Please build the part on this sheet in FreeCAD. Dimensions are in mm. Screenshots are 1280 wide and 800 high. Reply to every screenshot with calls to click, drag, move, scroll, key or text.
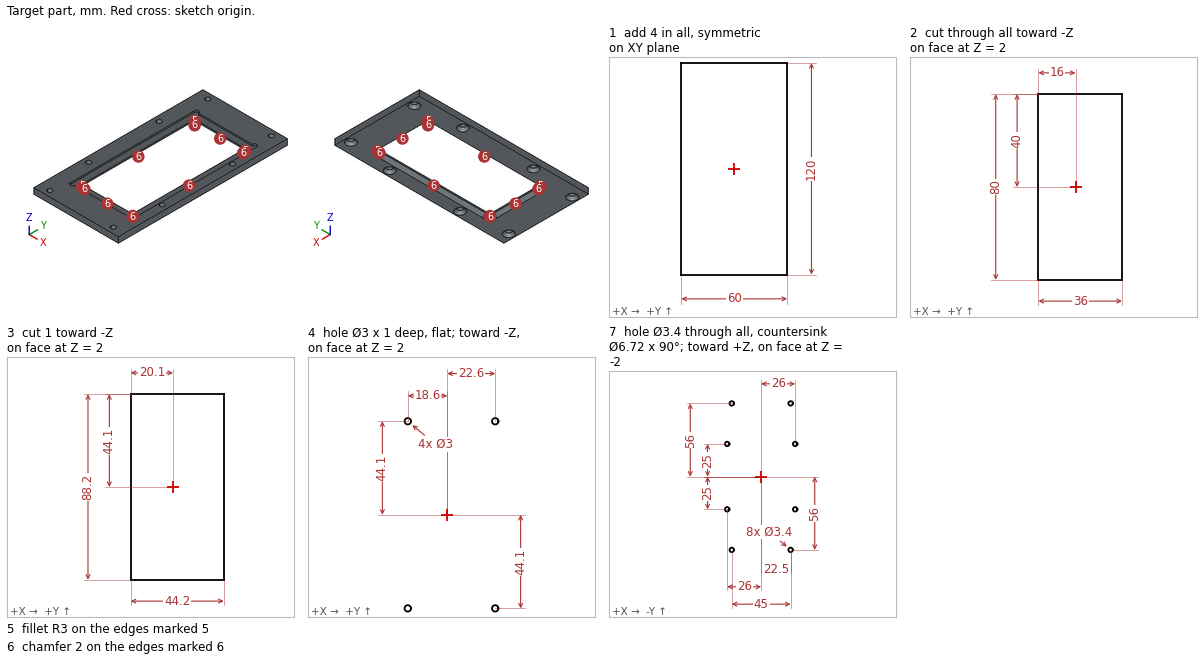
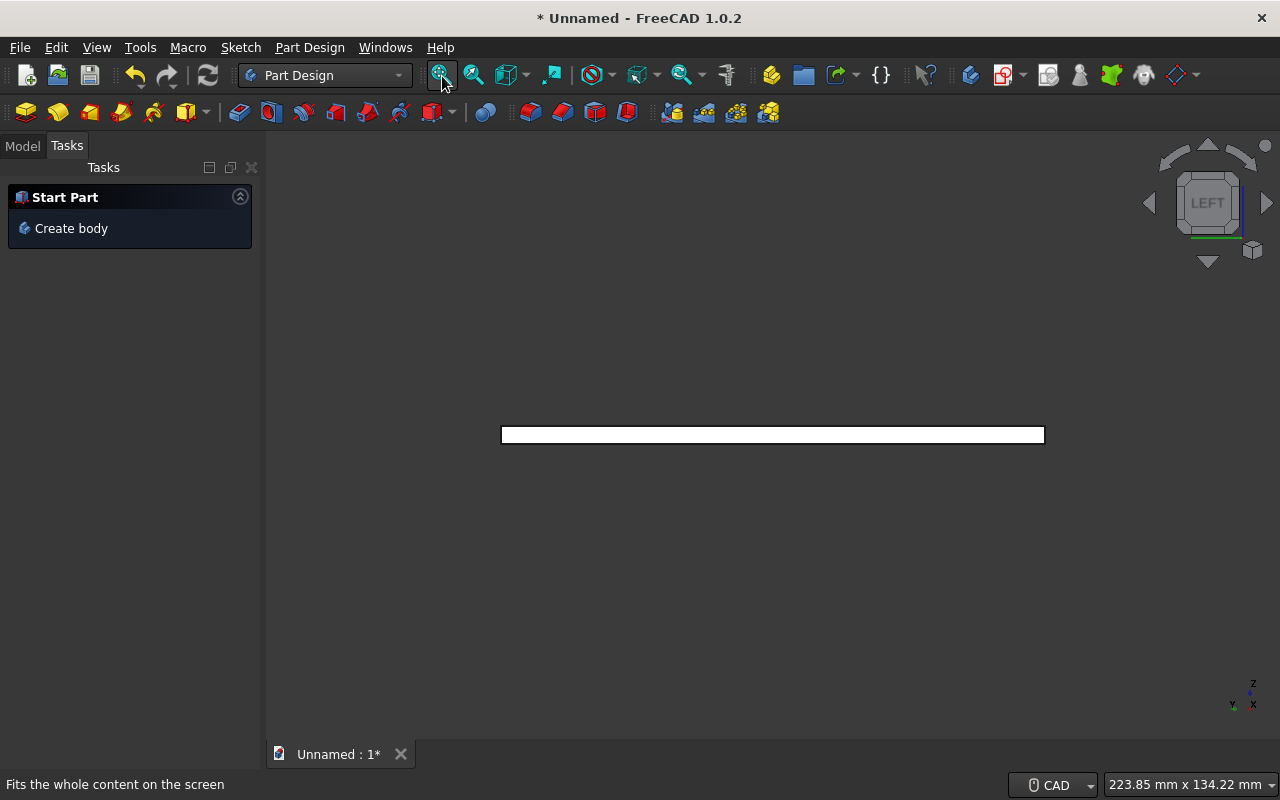
scroll(954, 436, up, 6)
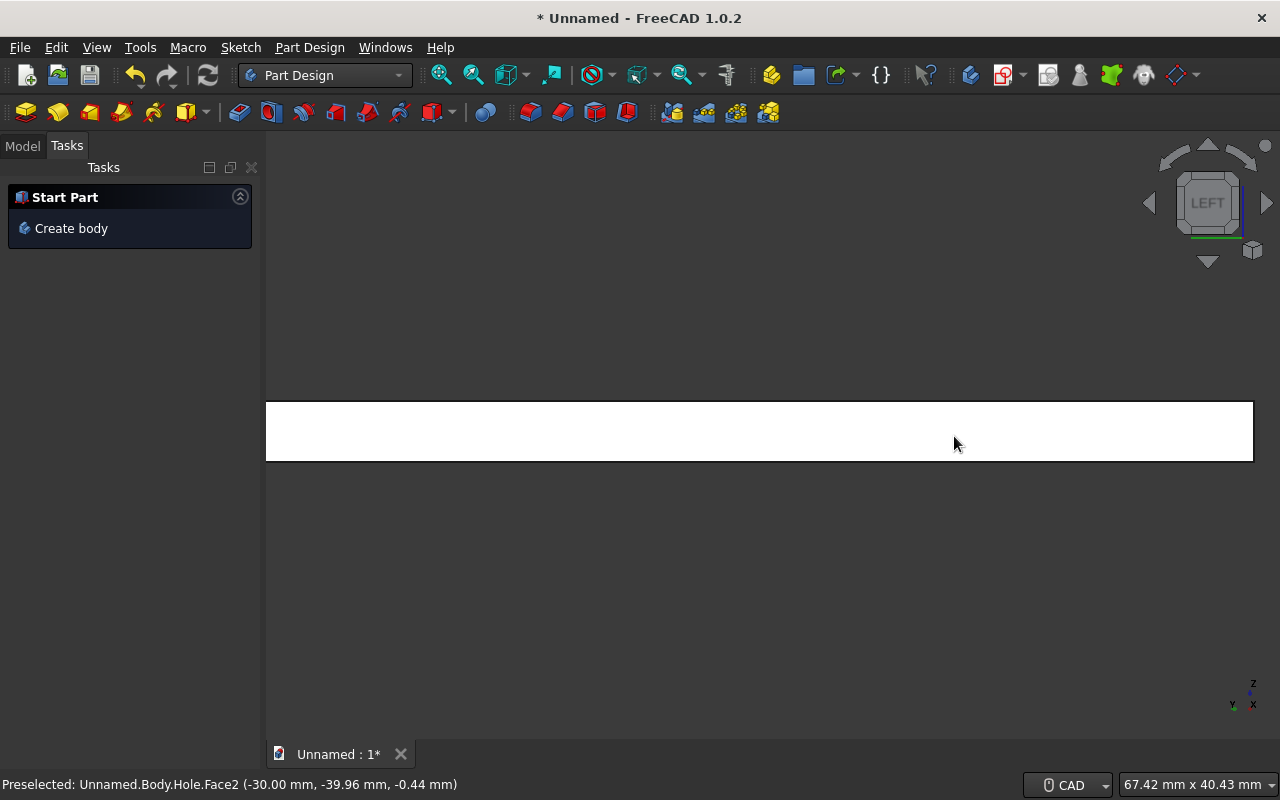
click(442, 76)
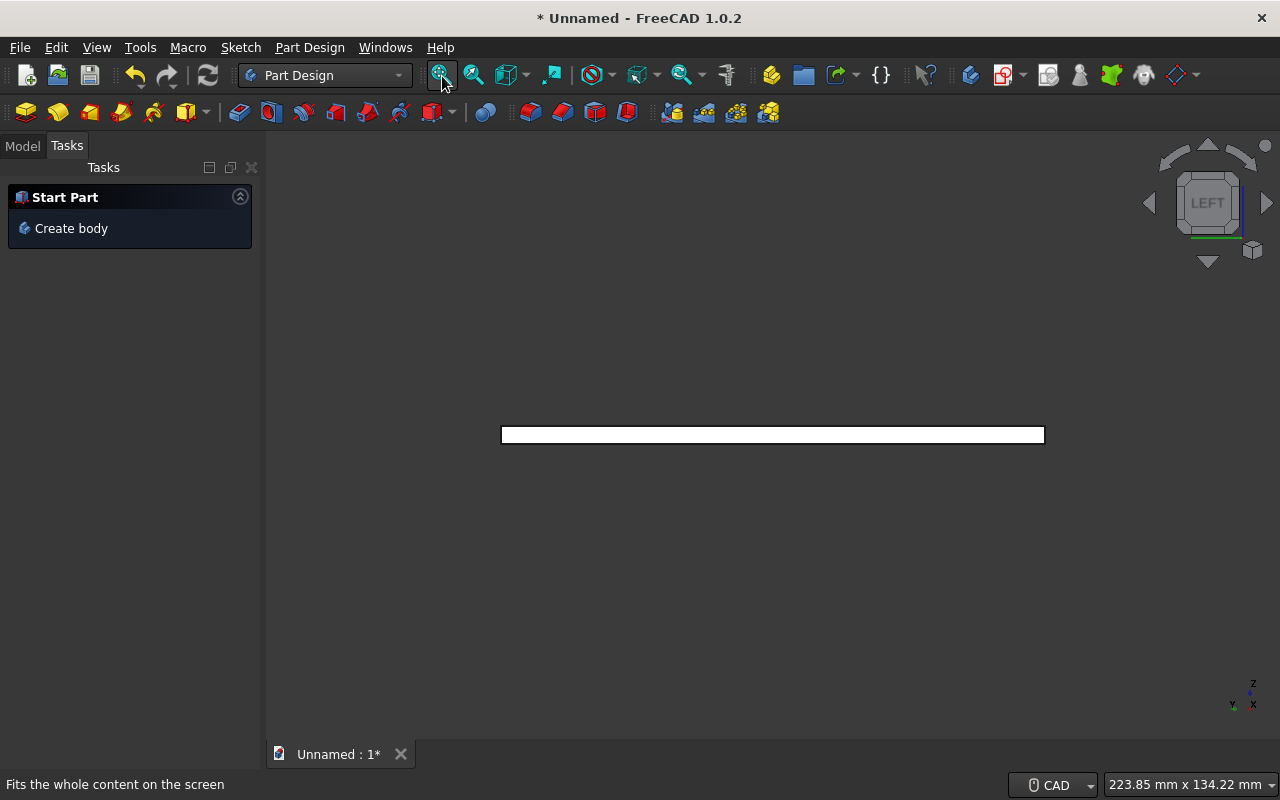
key(v)
key(3)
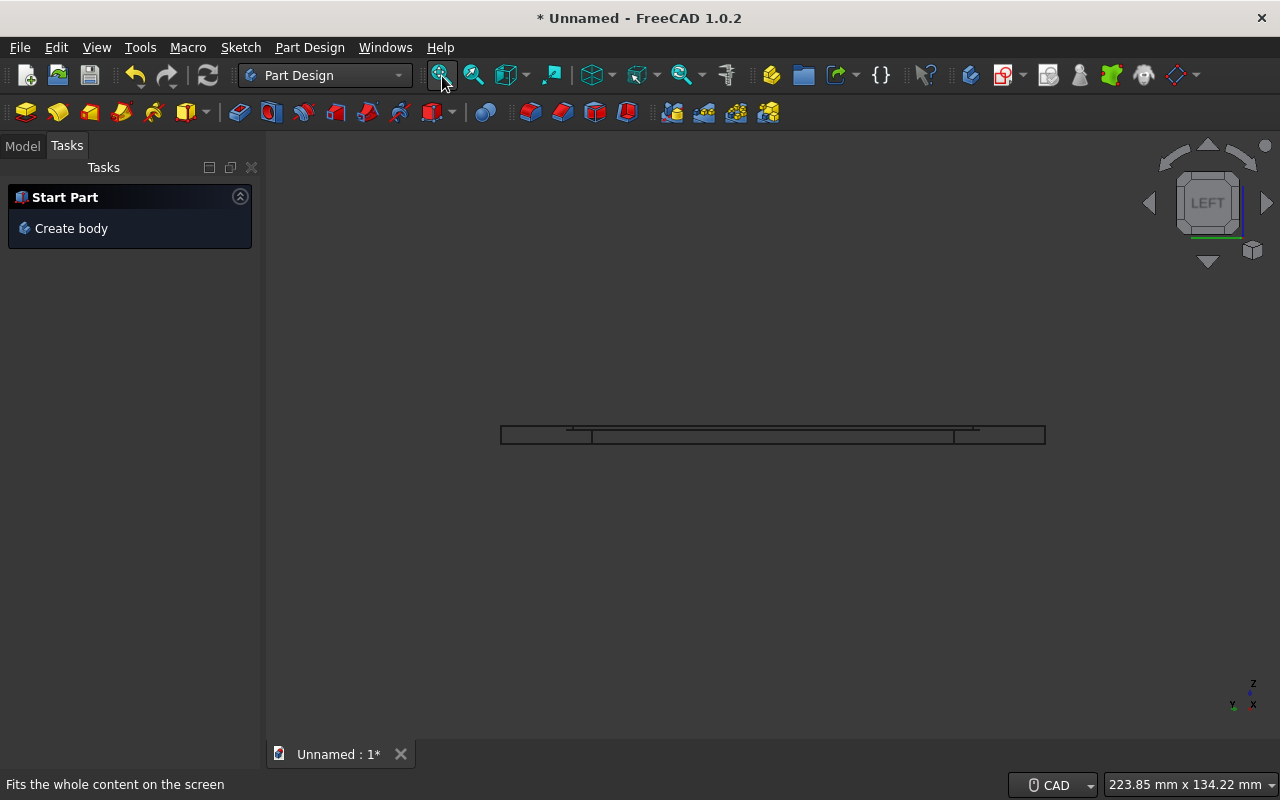
key(0)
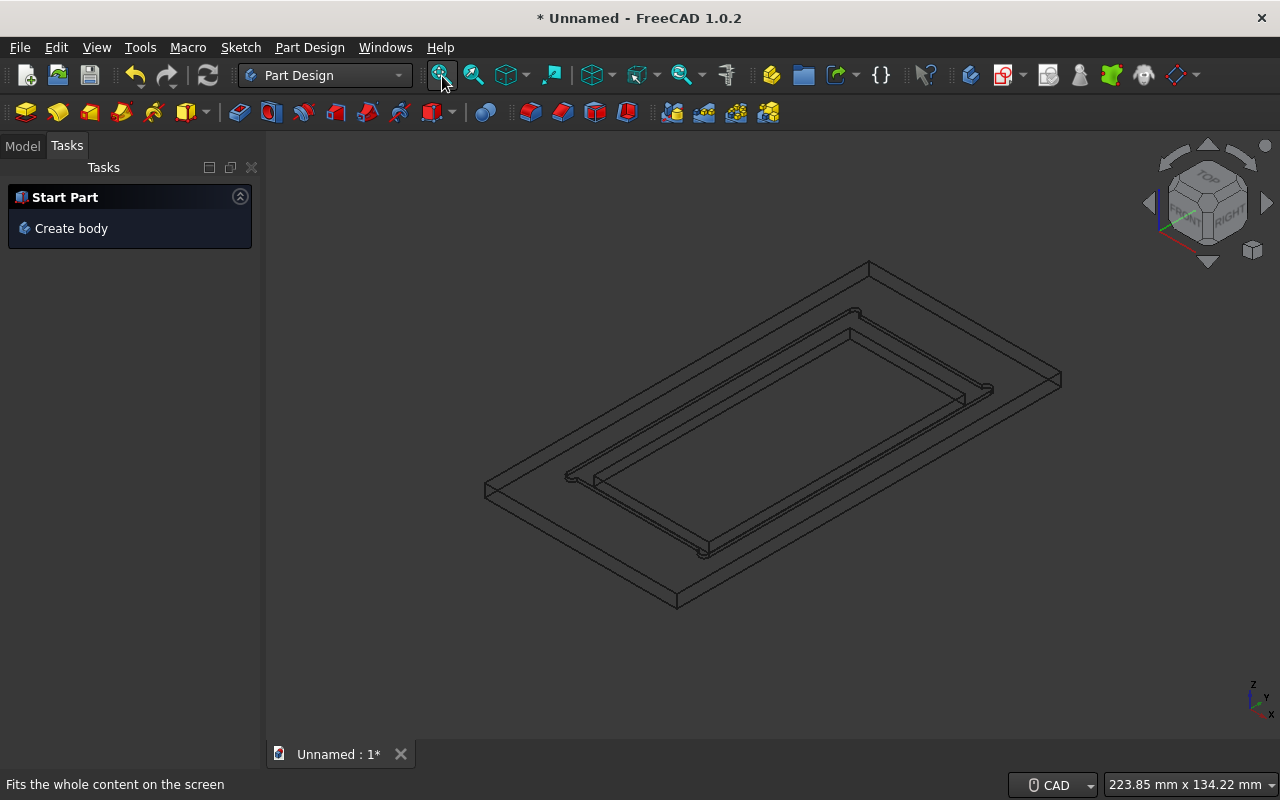
click(850, 335)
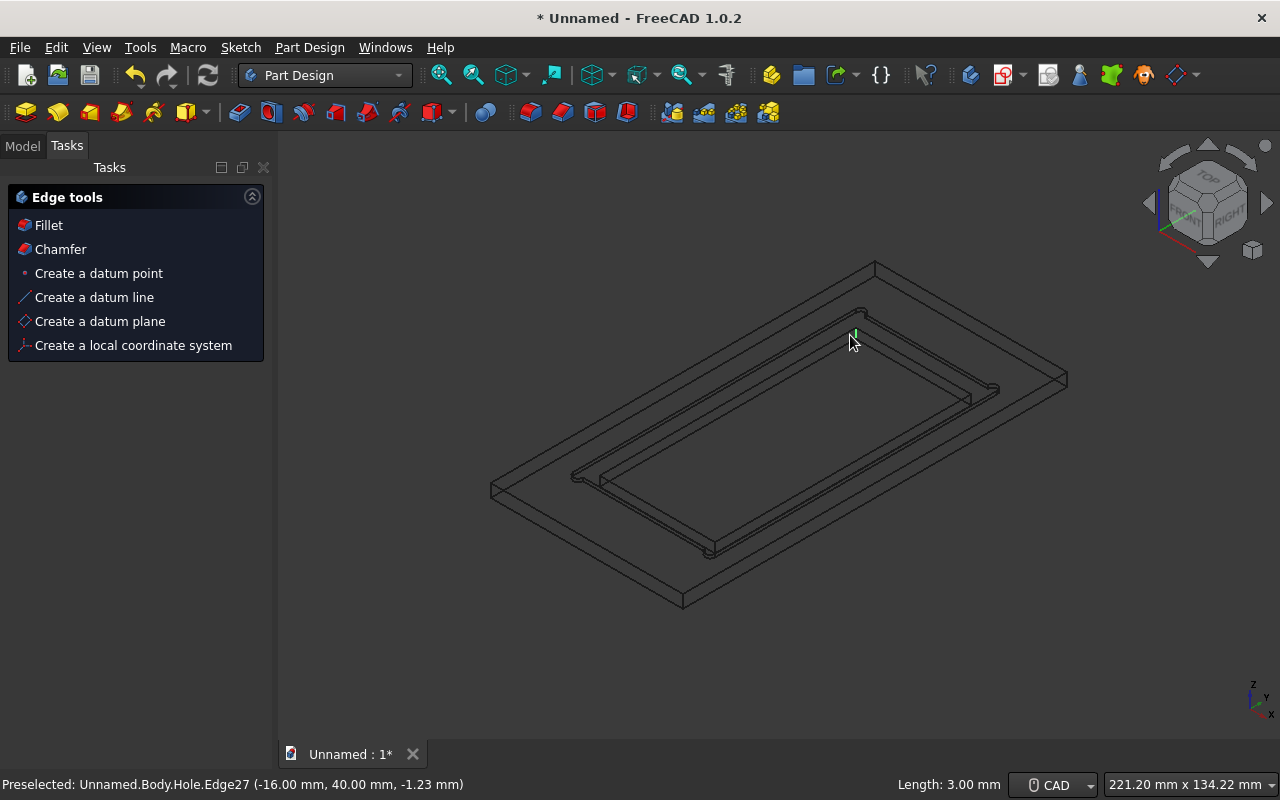
scroll(600, 480, up, 6)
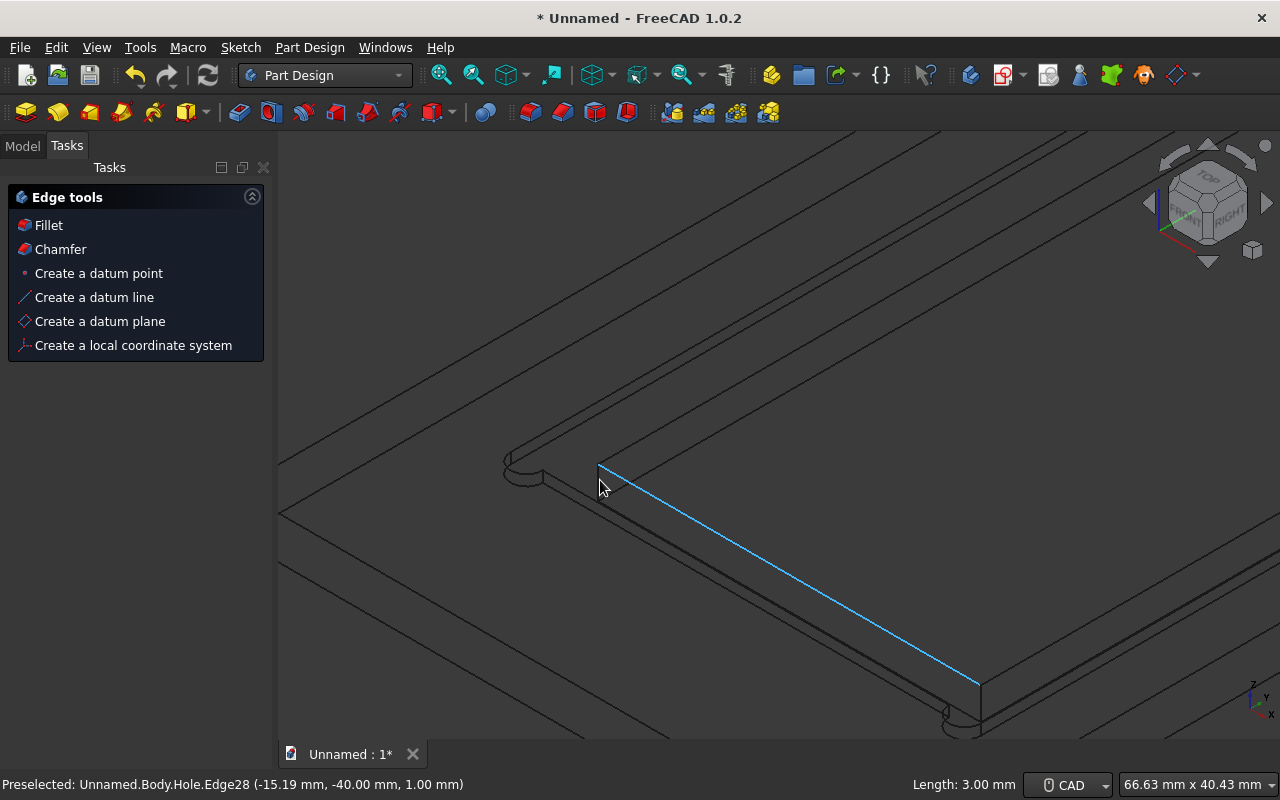
click(598, 482, ctrl)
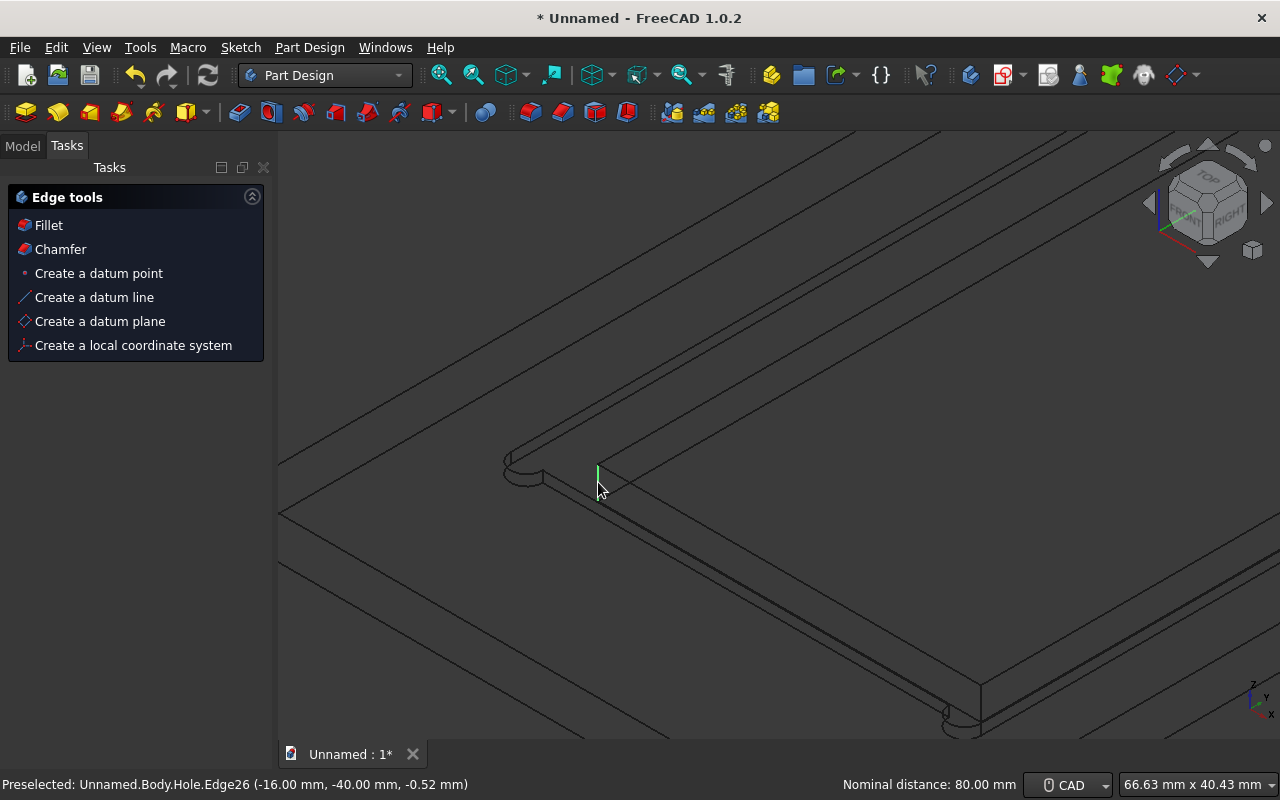
click(981, 703, ctrl)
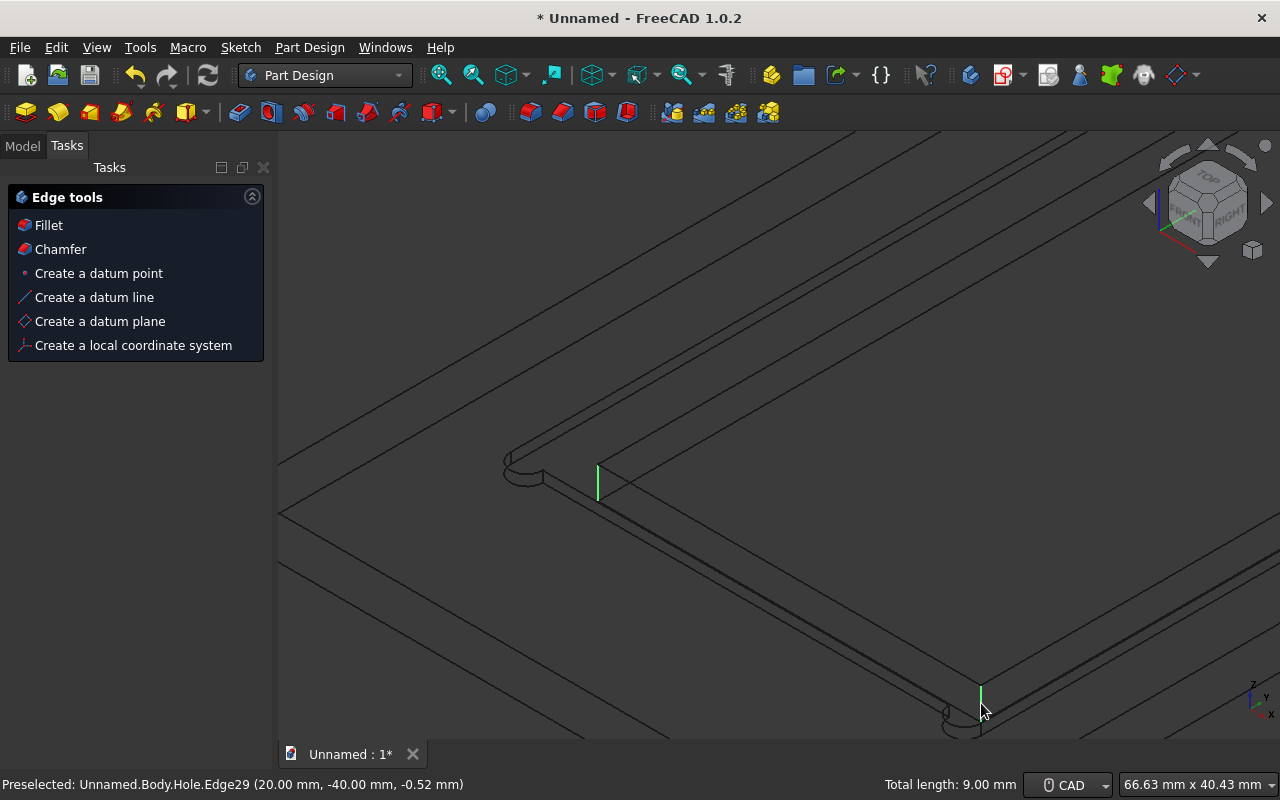
click(442, 76)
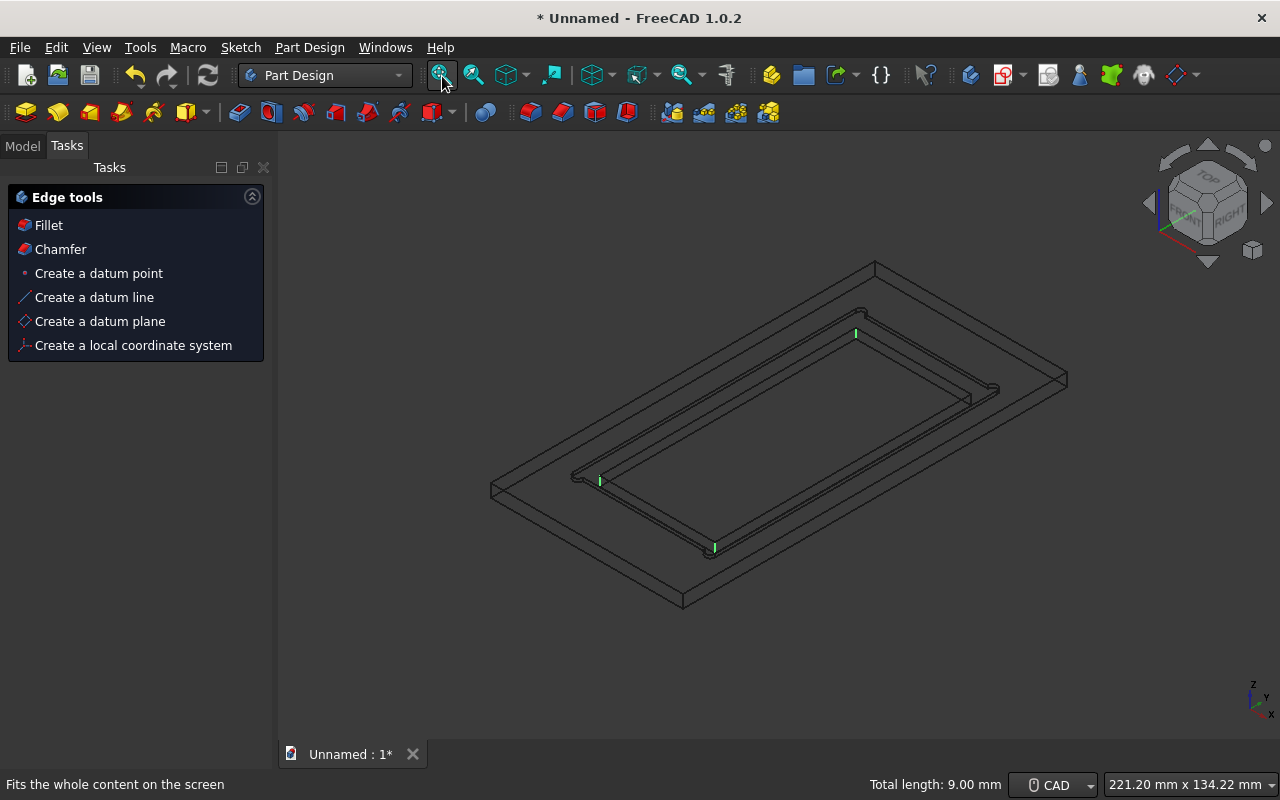
key(2)